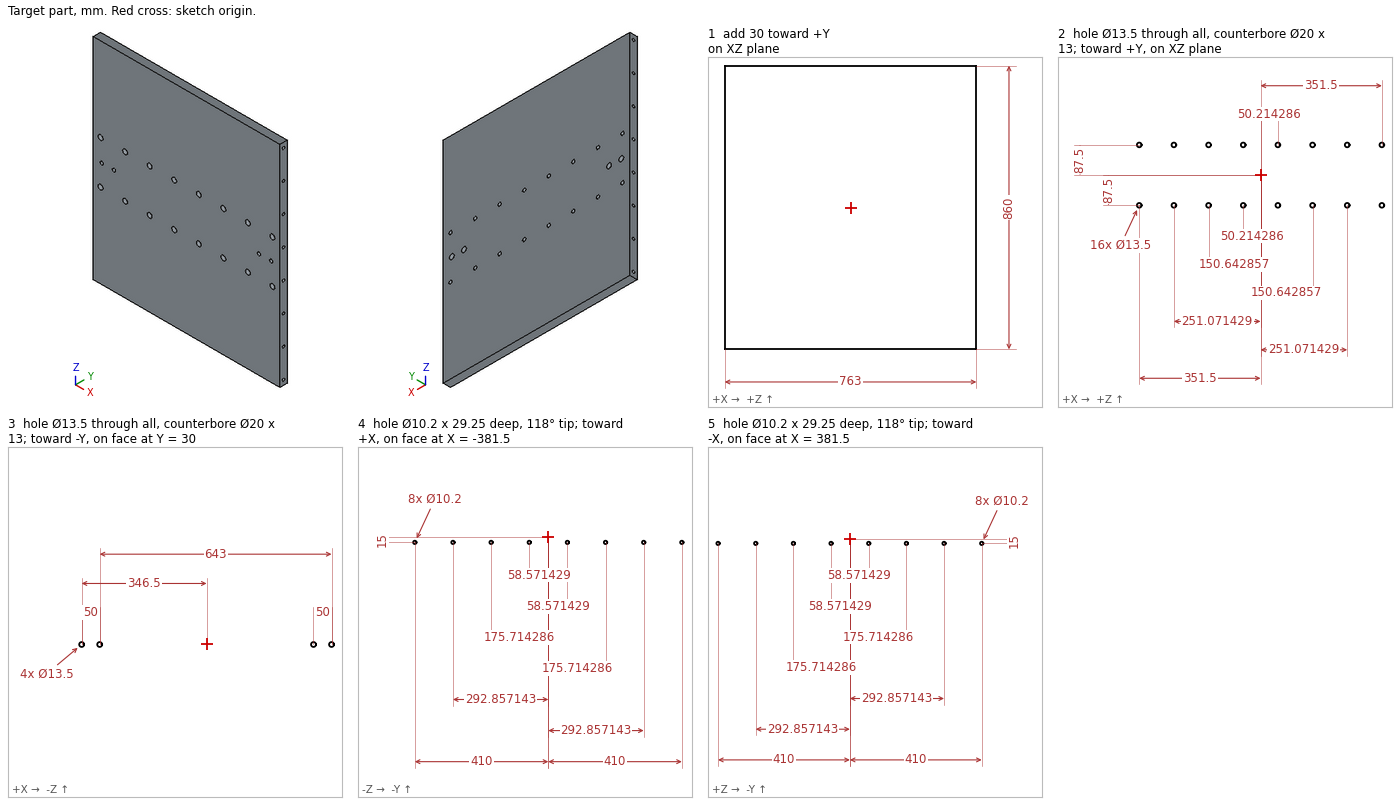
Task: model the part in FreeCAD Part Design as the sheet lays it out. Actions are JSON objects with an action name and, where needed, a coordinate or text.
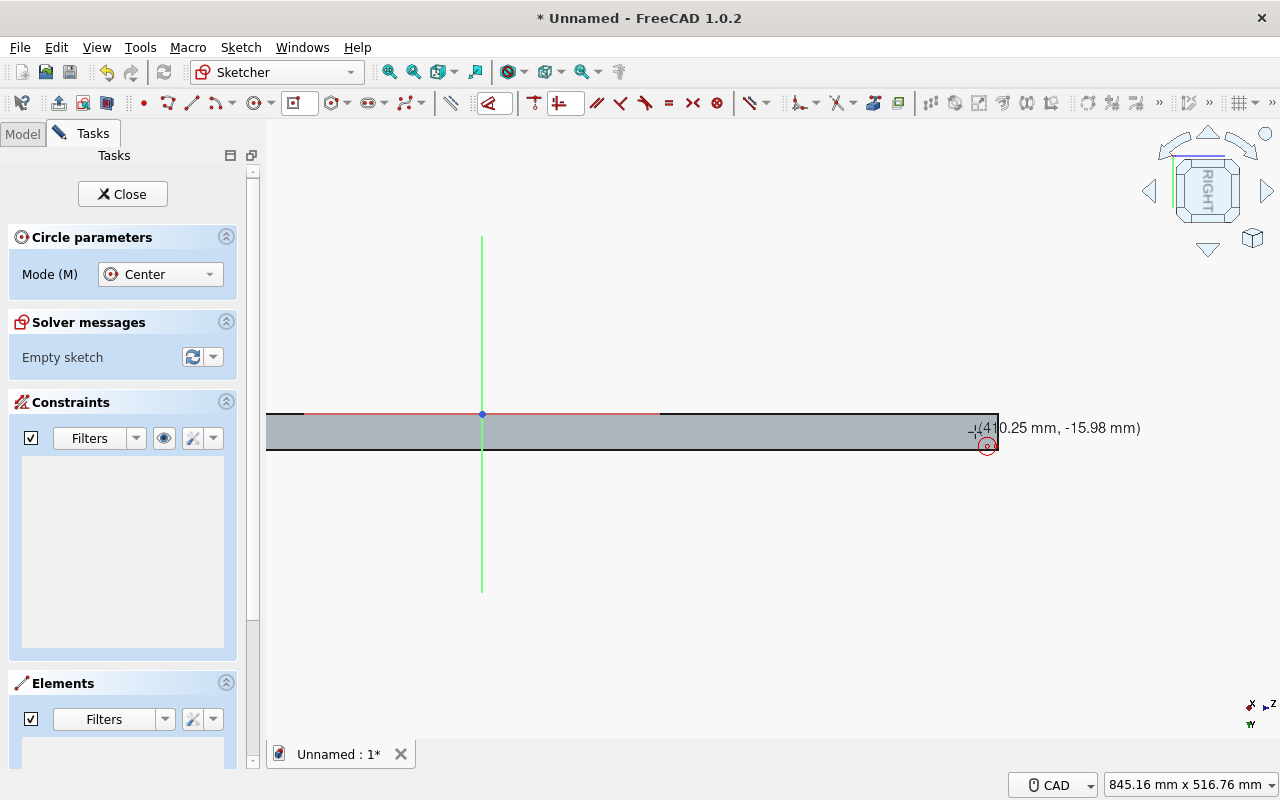
{"action": "left_click", "coordinate": [974, 432]}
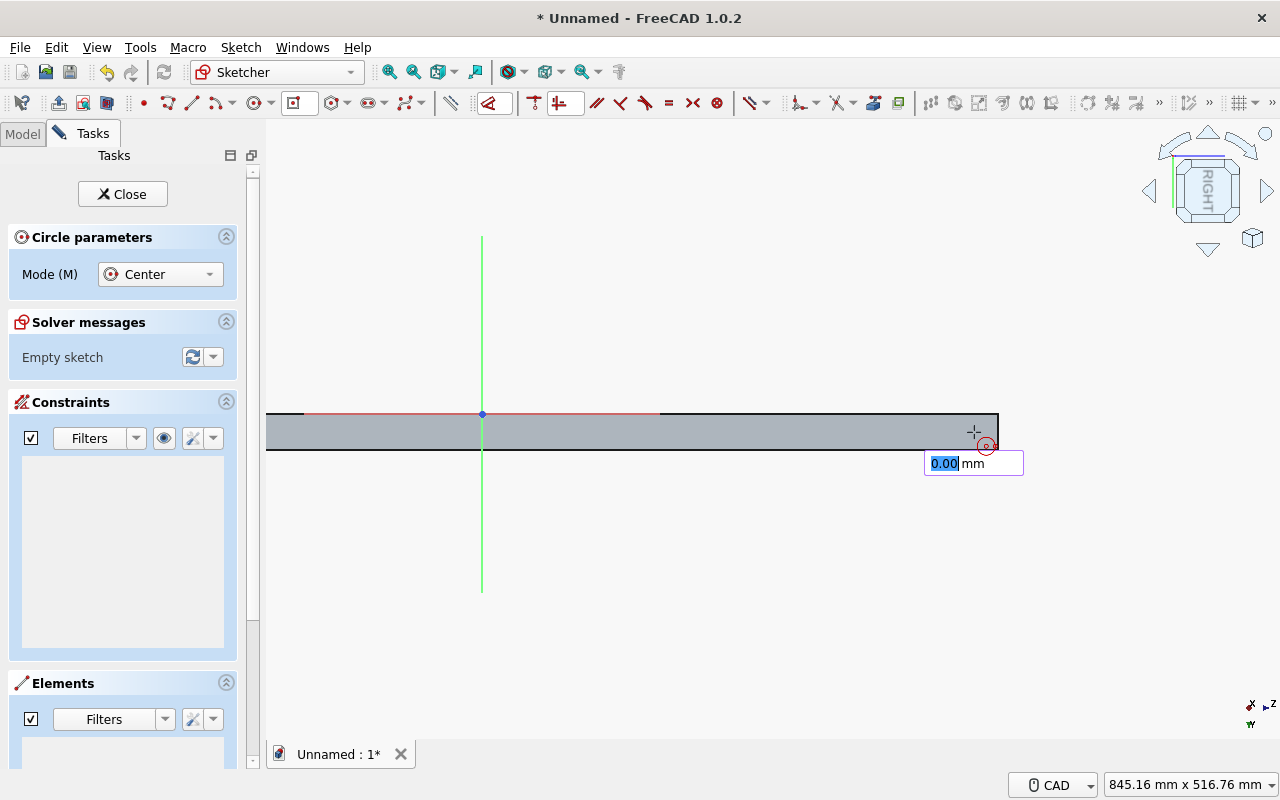
{"action": "scroll", "coordinate": [978, 437], "scroll_direction": "up", "scroll_amount": 5}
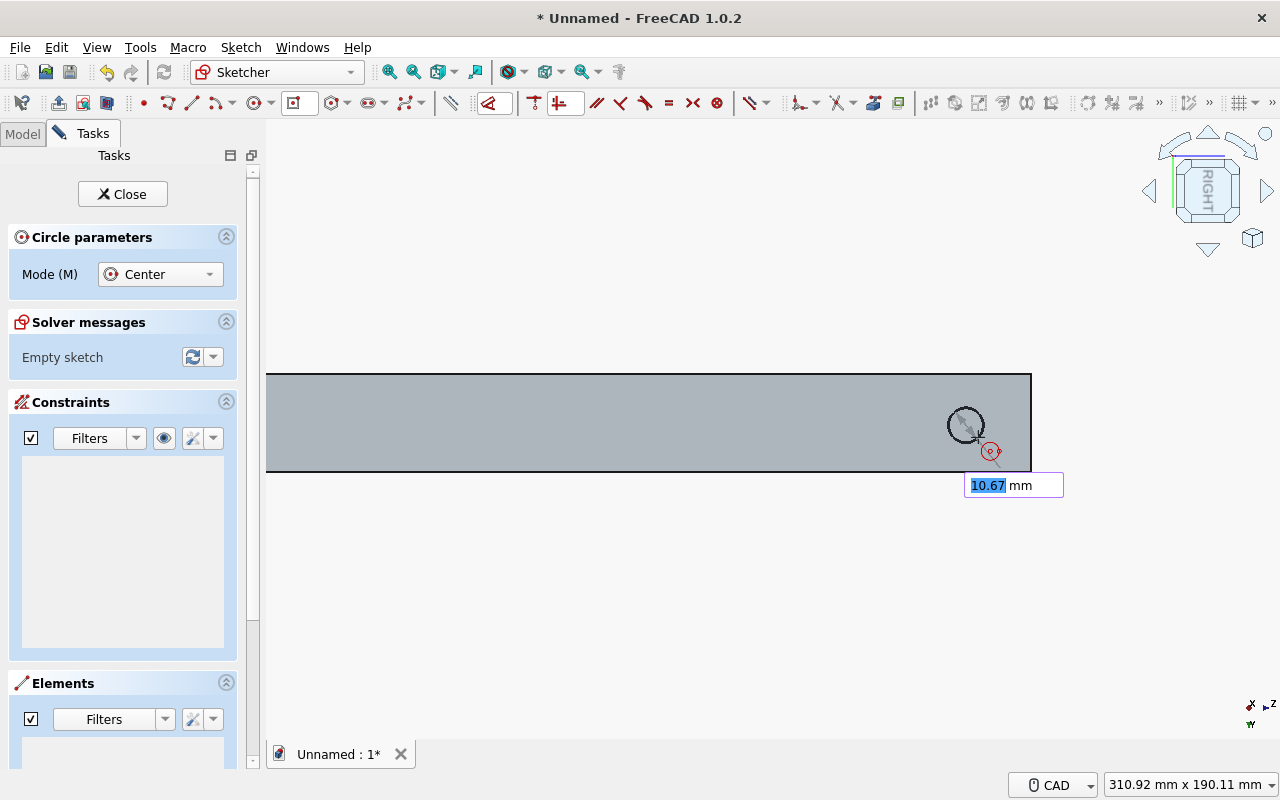
{"action": "left_click", "coordinate": [978, 435]}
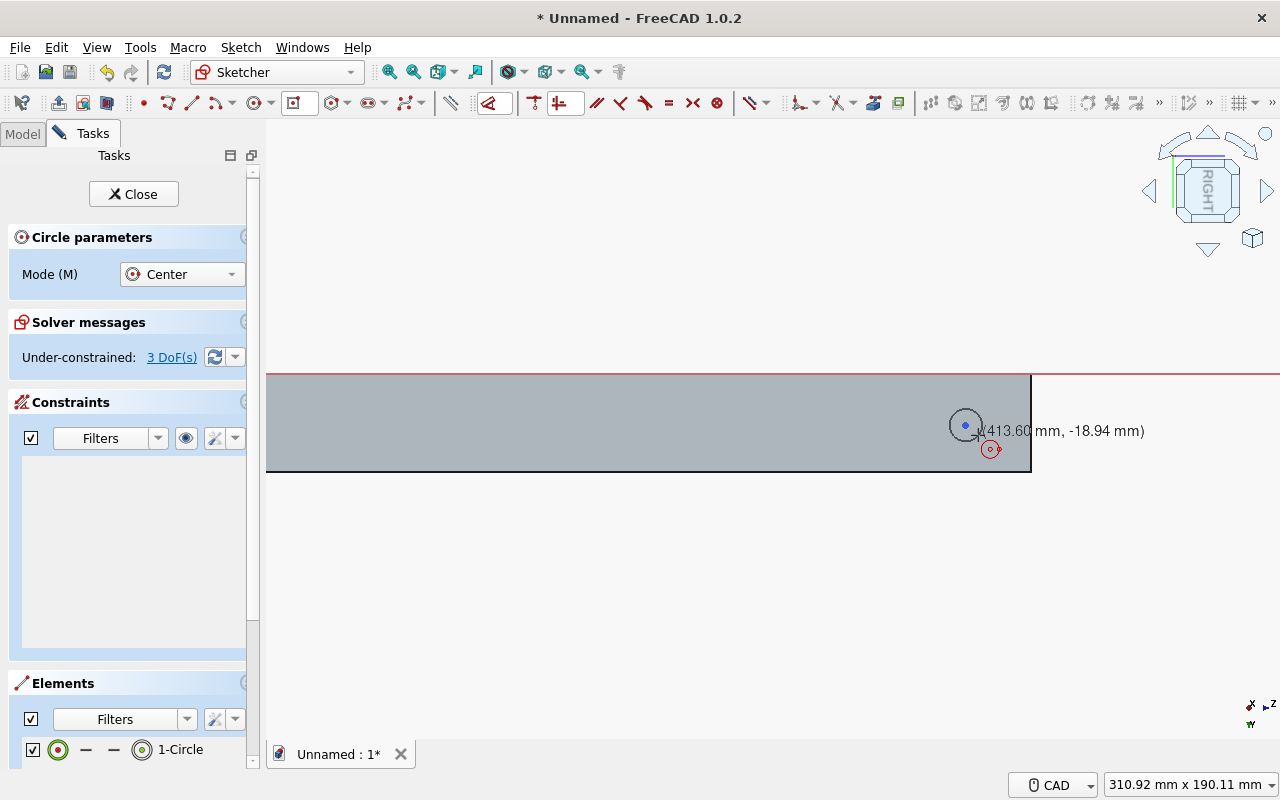
{"action": "scroll", "coordinate": [584, 423], "scroll_direction": "up", "scroll_amount": 2}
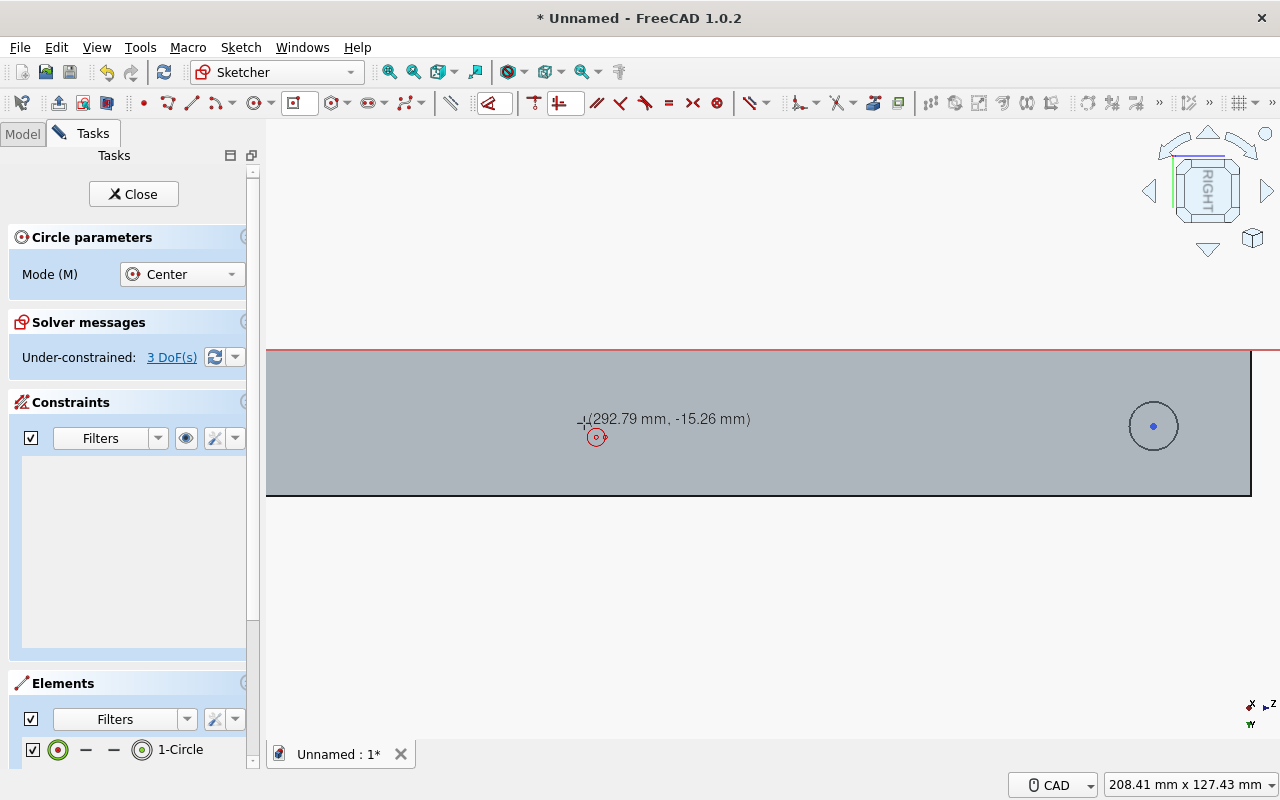
{"action": "scroll", "coordinate": [946, 434], "scroll_direction": "down", "scroll_amount": 10}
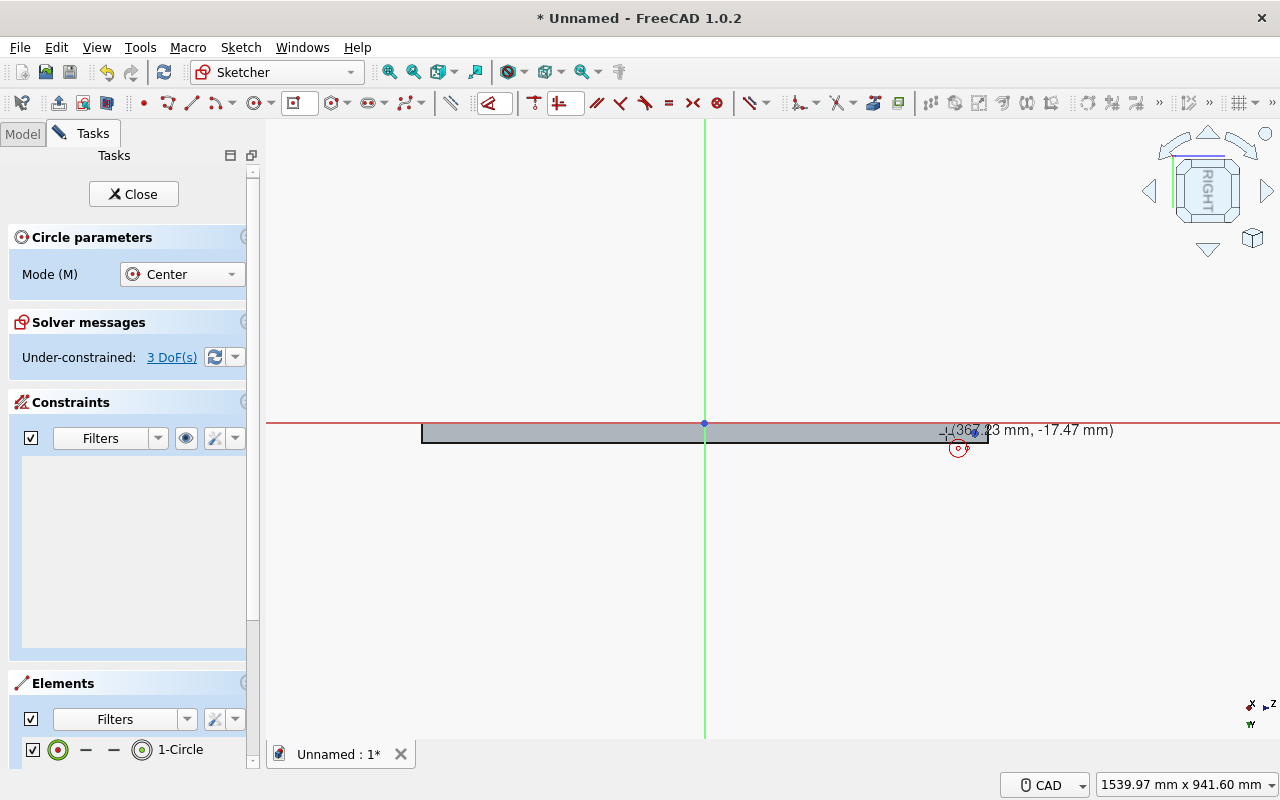
{"action": "scroll", "coordinate": [898, 433], "scroll_direction": "up", "scroll_amount": 3}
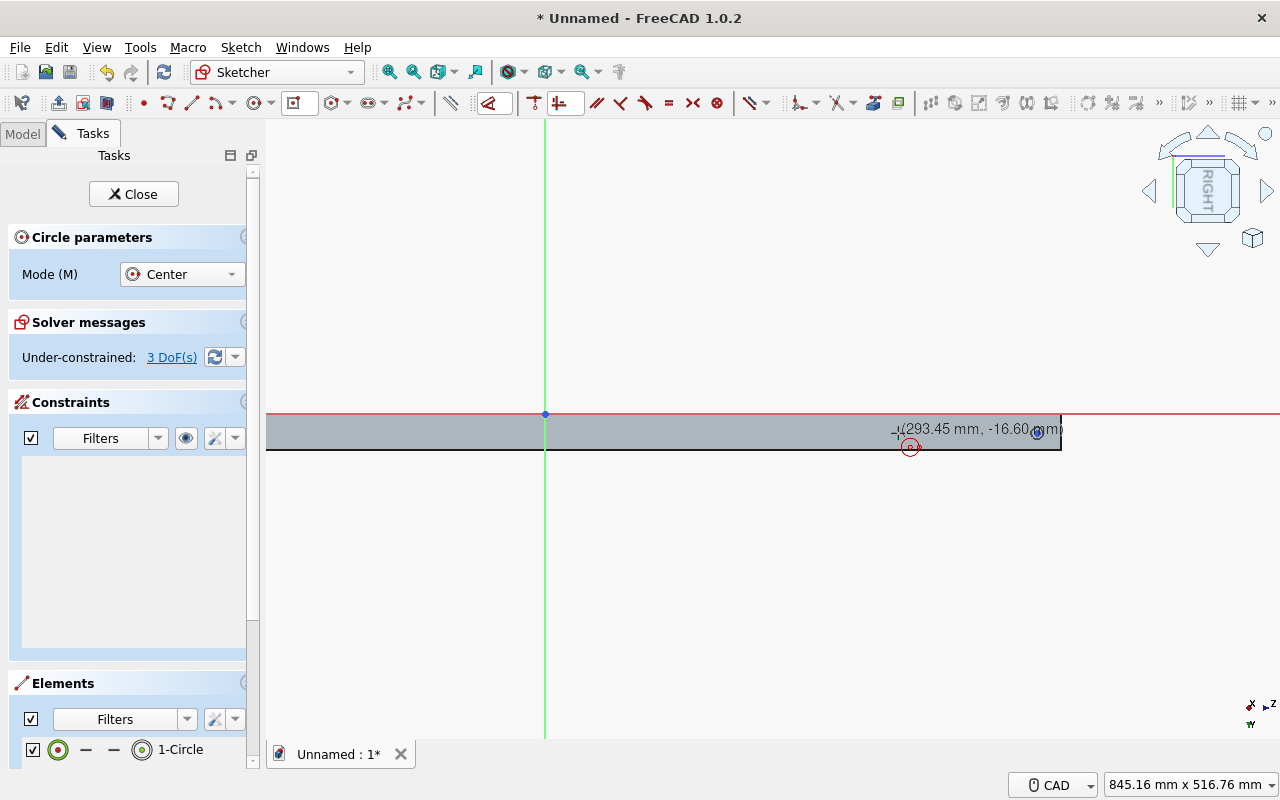
{"action": "left_click", "coordinate": [897, 432]}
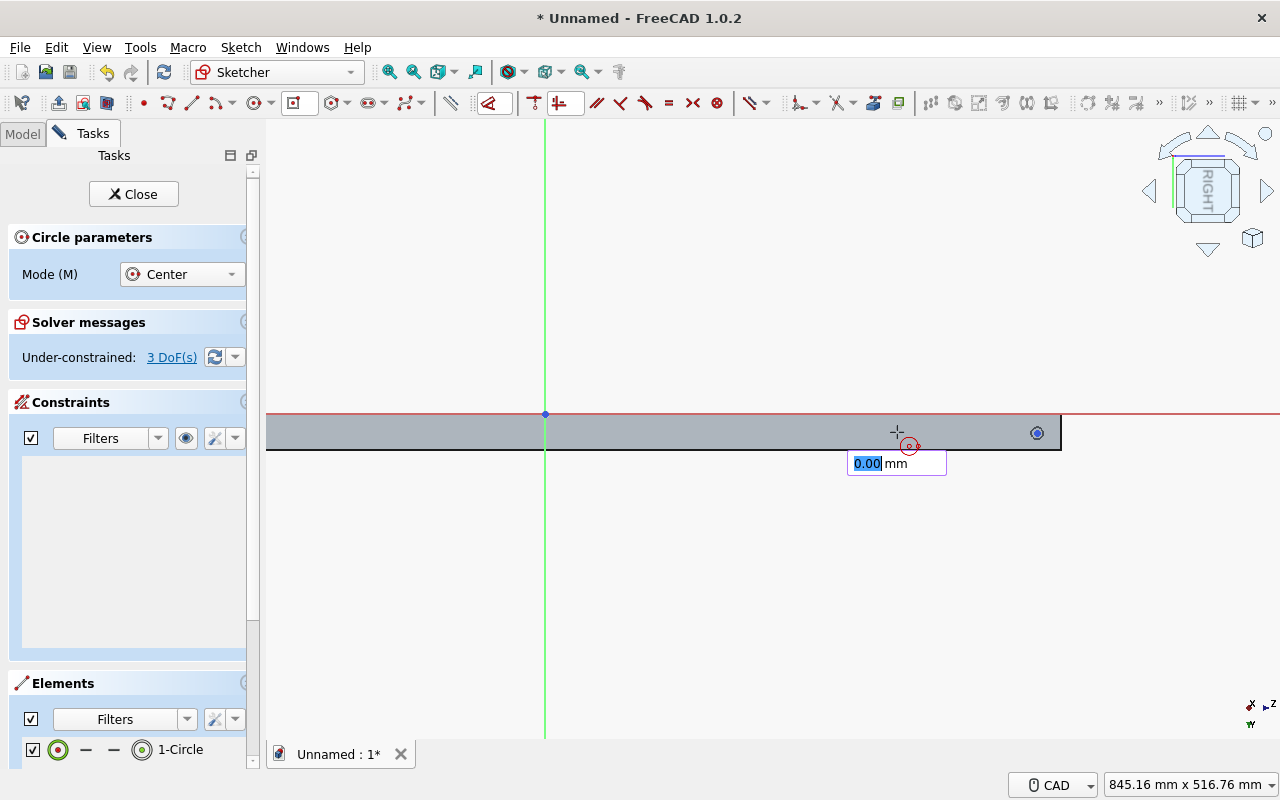
{"action": "scroll", "coordinate": [901, 437], "scroll_direction": "up", "scroll_amount": 5}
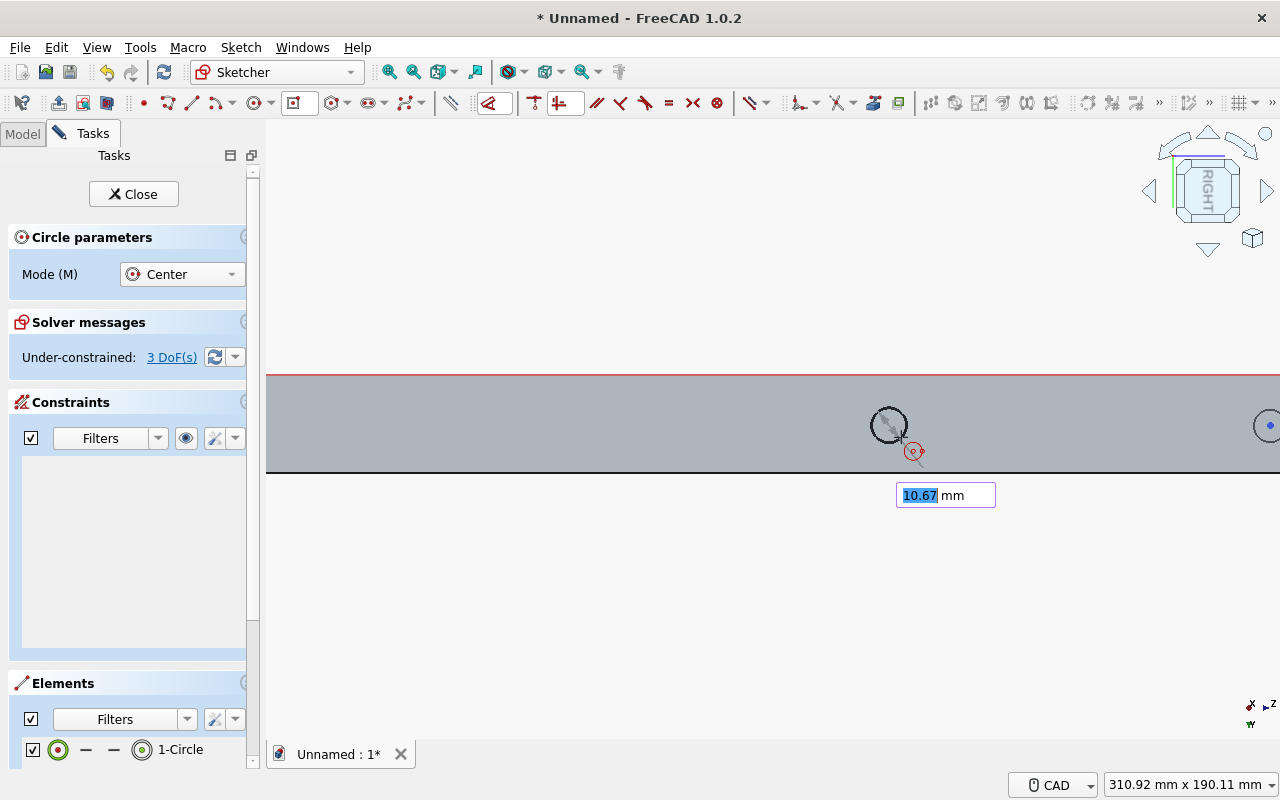
{"action": "left_click", "coordinate": [900, 436]}